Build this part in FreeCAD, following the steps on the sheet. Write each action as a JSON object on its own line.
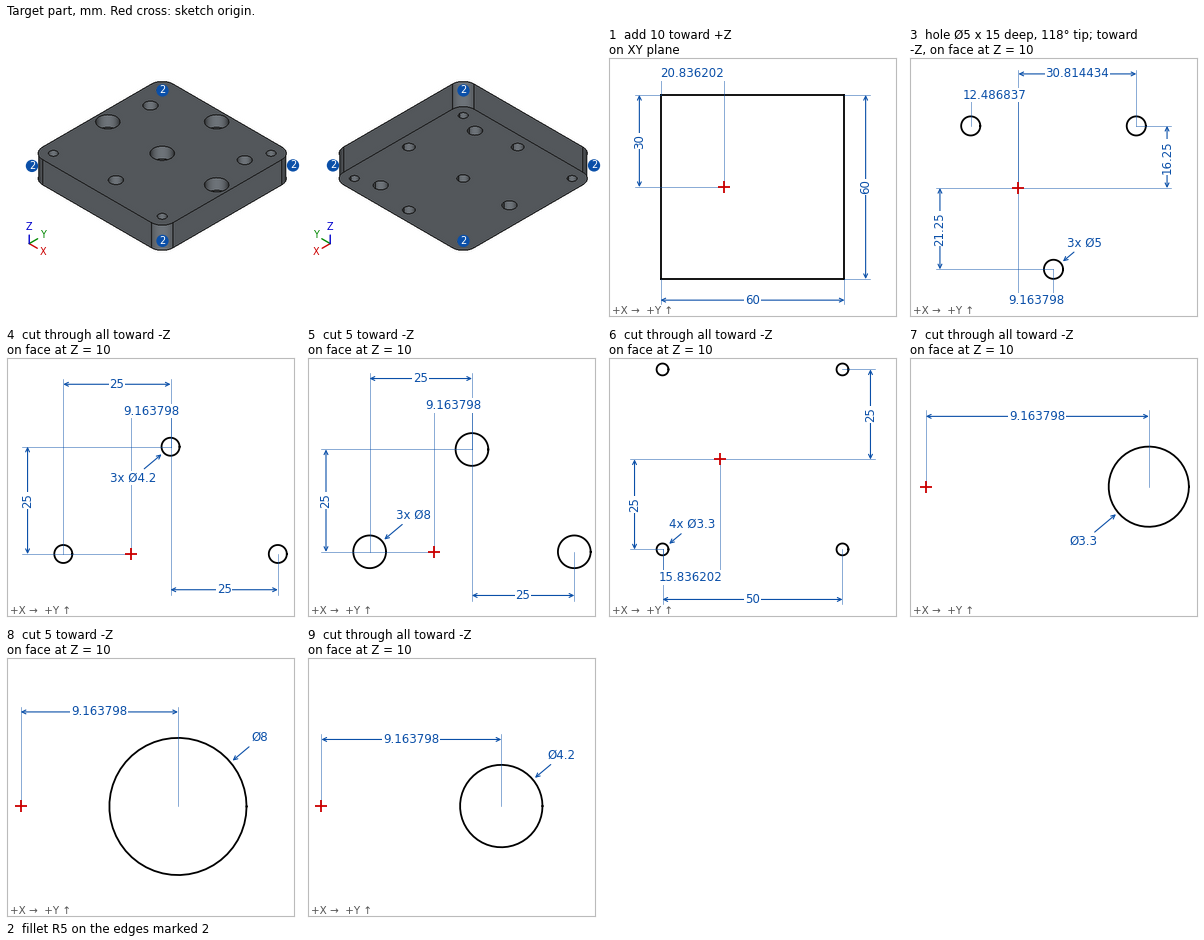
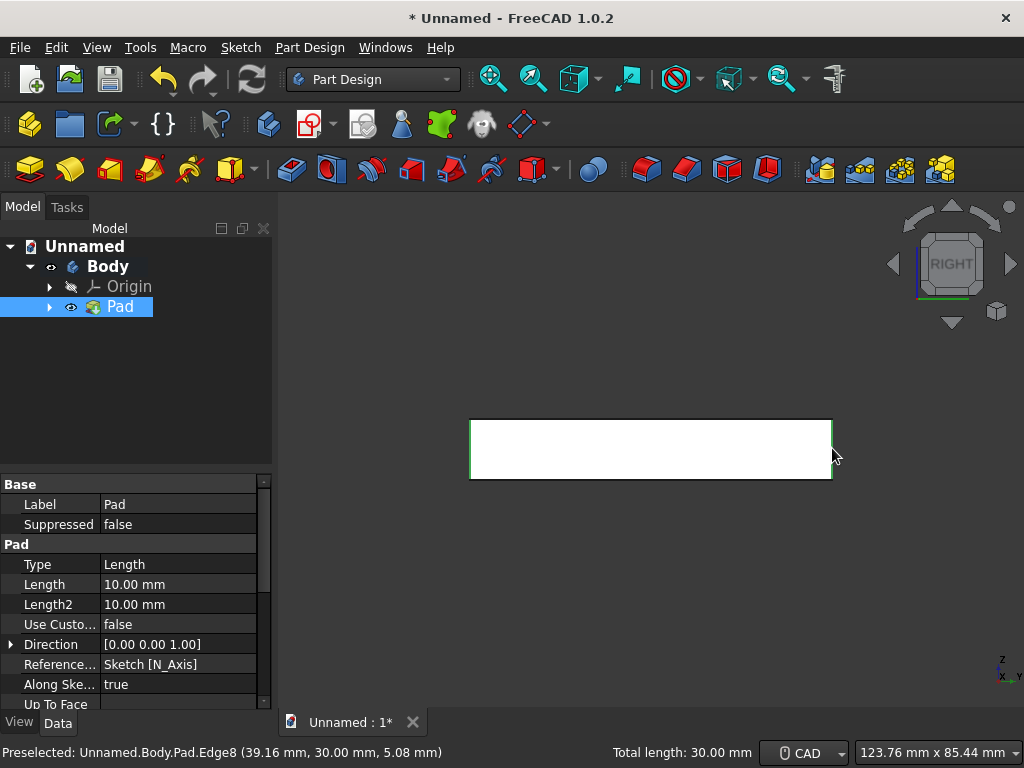
{"action": "key", "text": "5"}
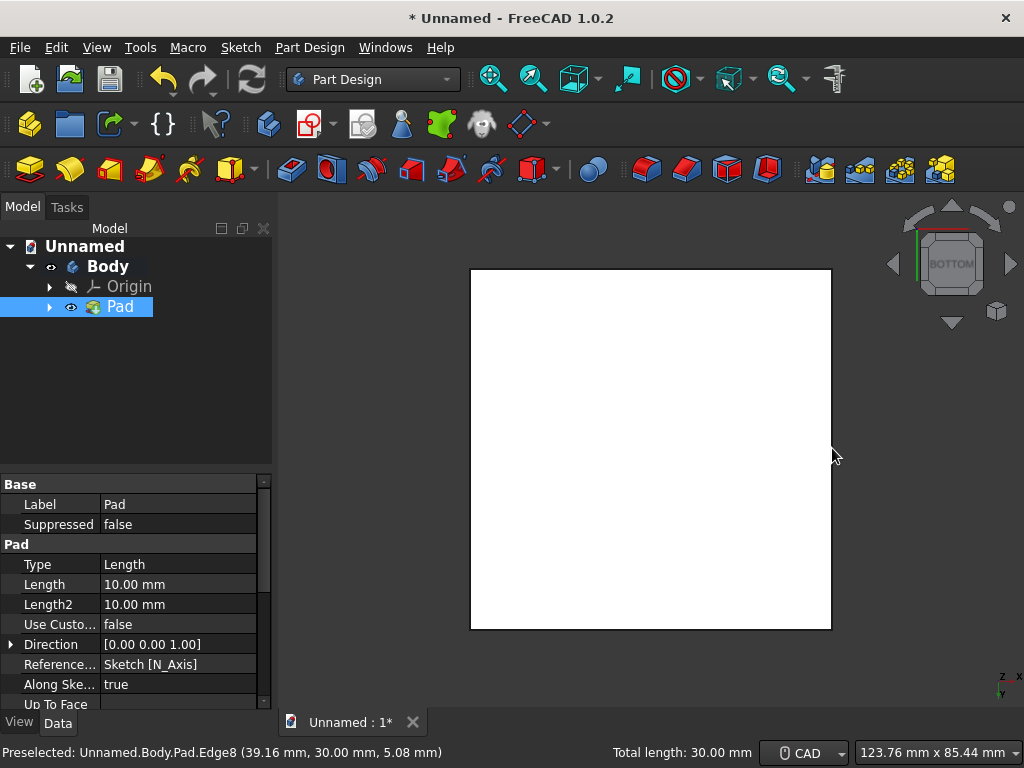
{"action": "key", "text": "4"}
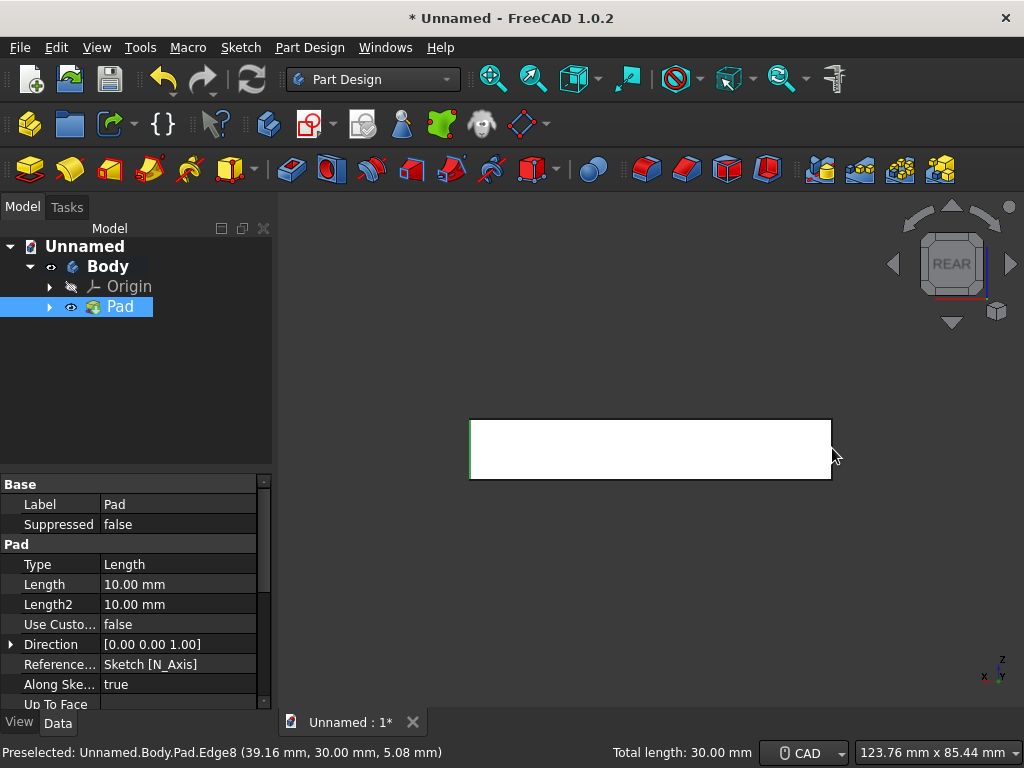
{"action": "left_click", "coordinate": [832, 449], "text": "ctrl"}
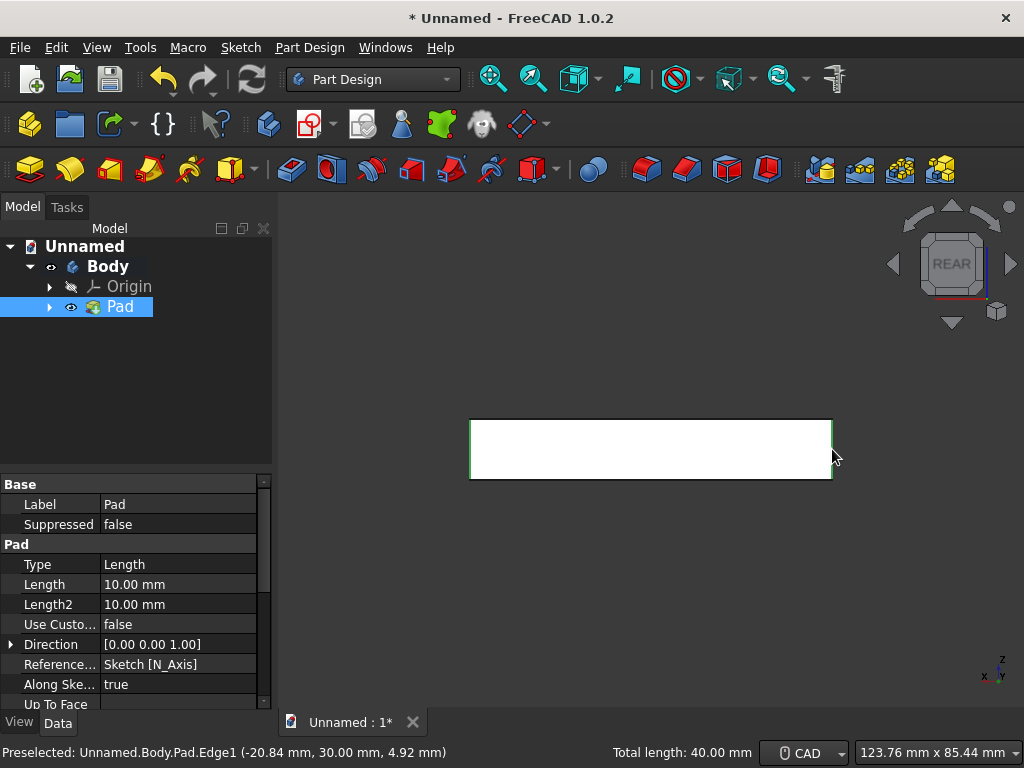
{"action": "left_click", "coordinate": [648, 170]}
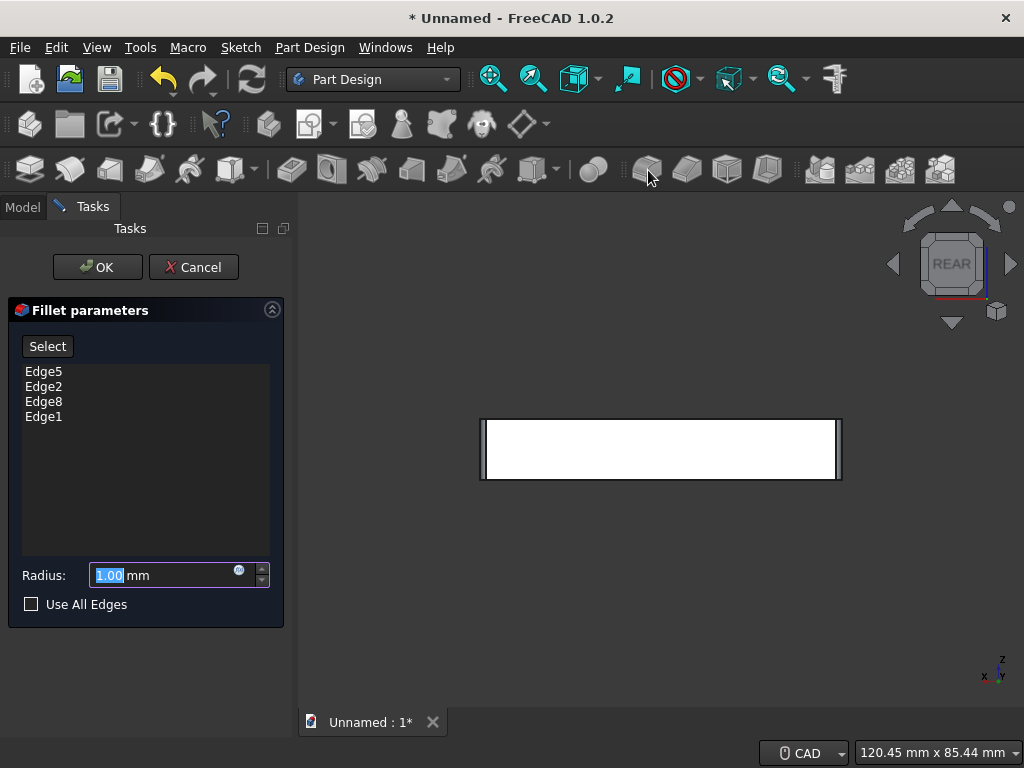
{"action": "type", "text": "5"}
{"action": "key", "text": "Tab"}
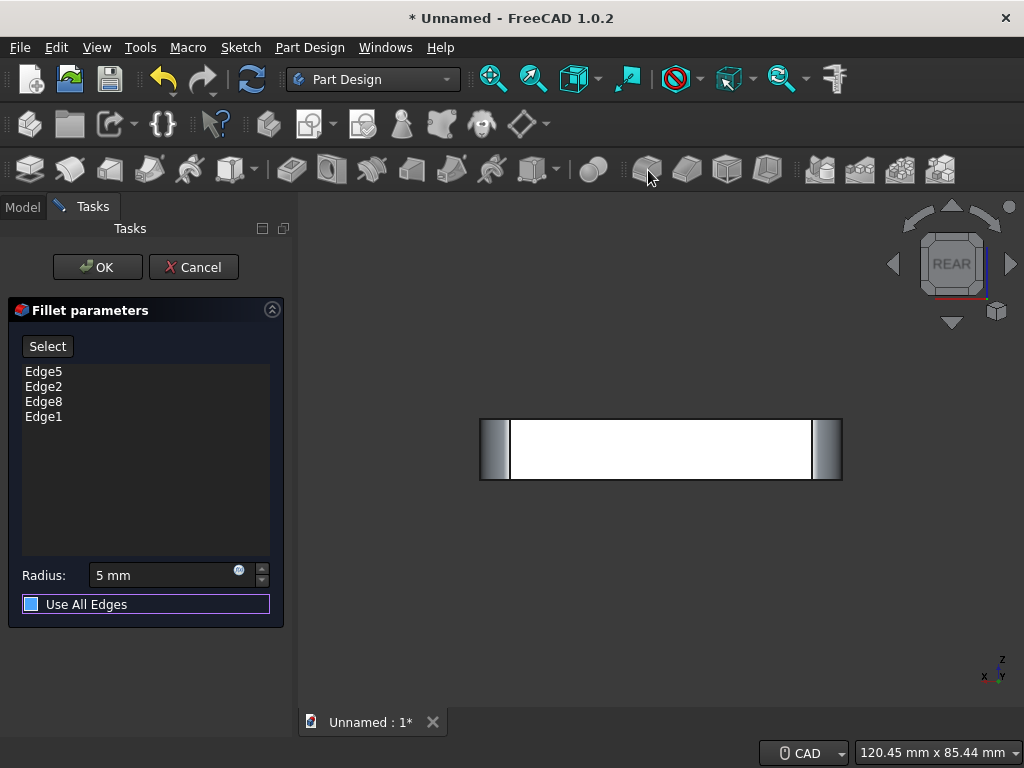
{"action": "left_click", "coordinate": [98, 267]}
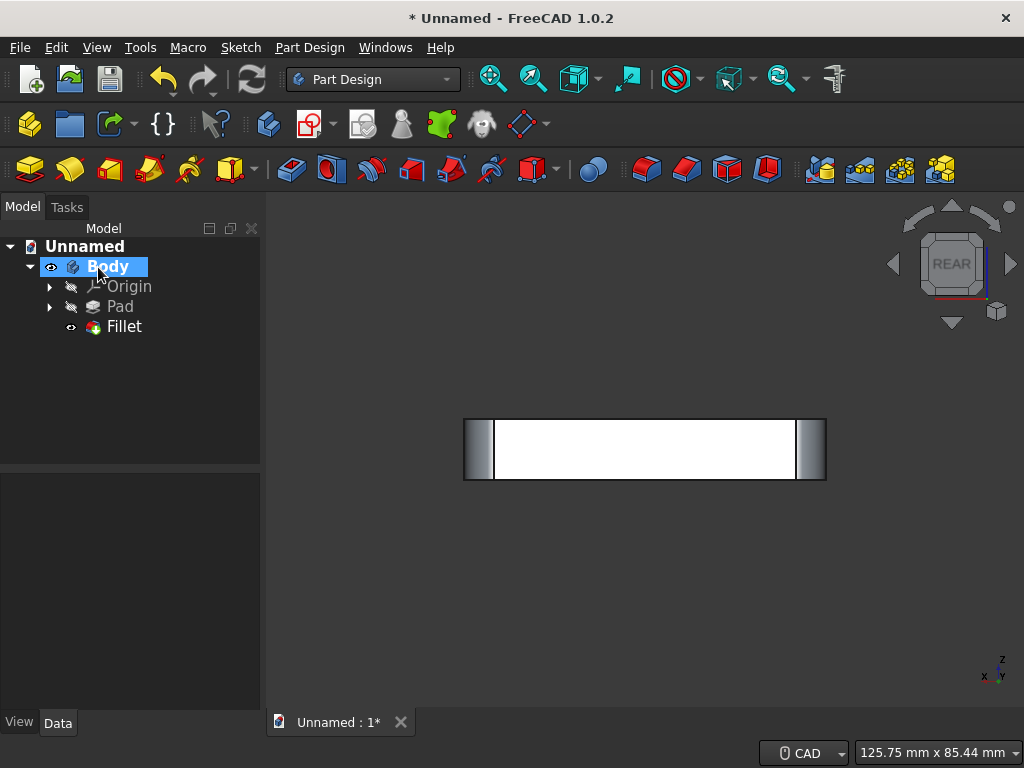
{"action": "key", "text": "0"}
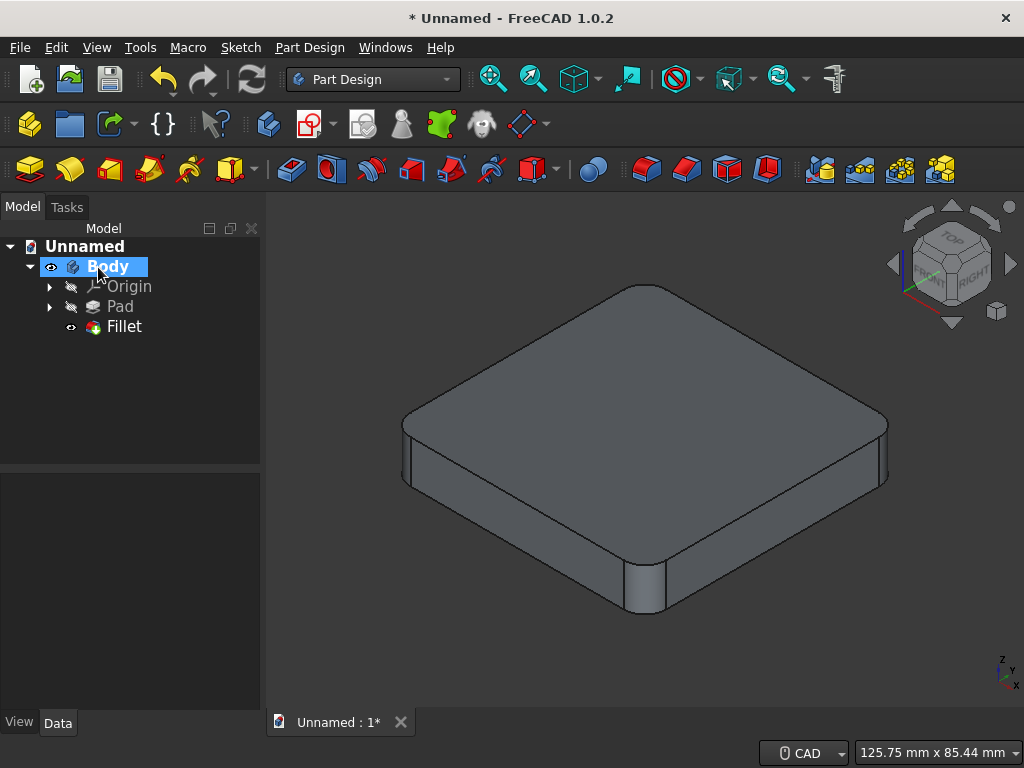
{"action": "left_click", "coordinate": [645, 424]}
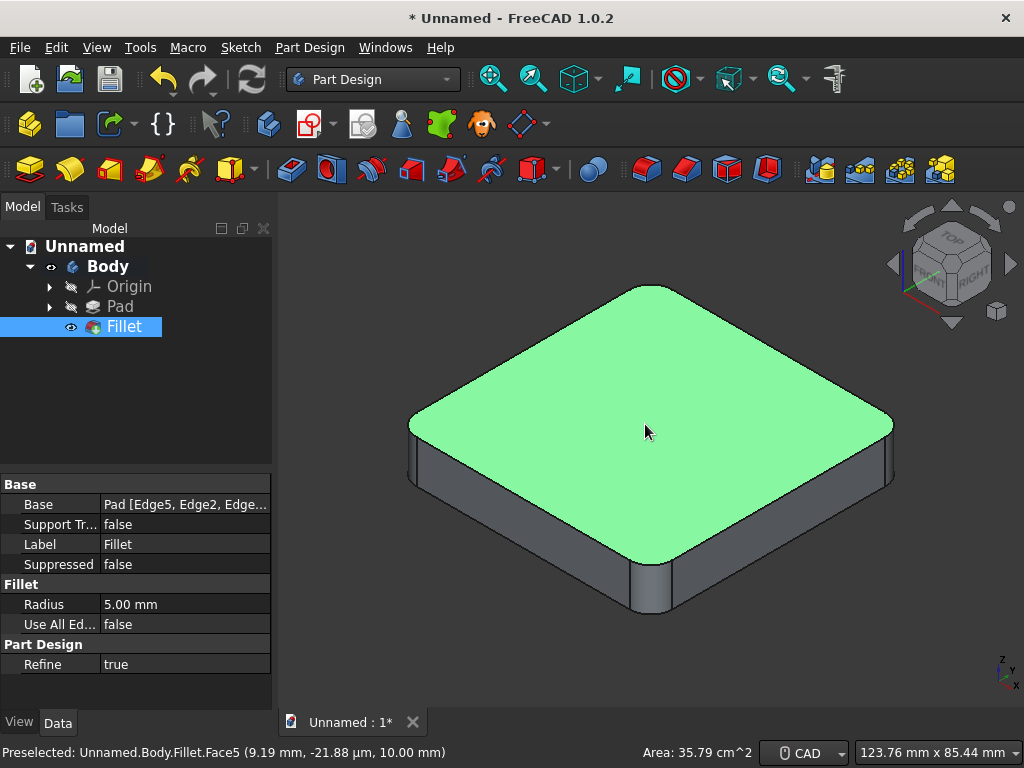
{"action": "left_click", "coordinate": [310, 124]}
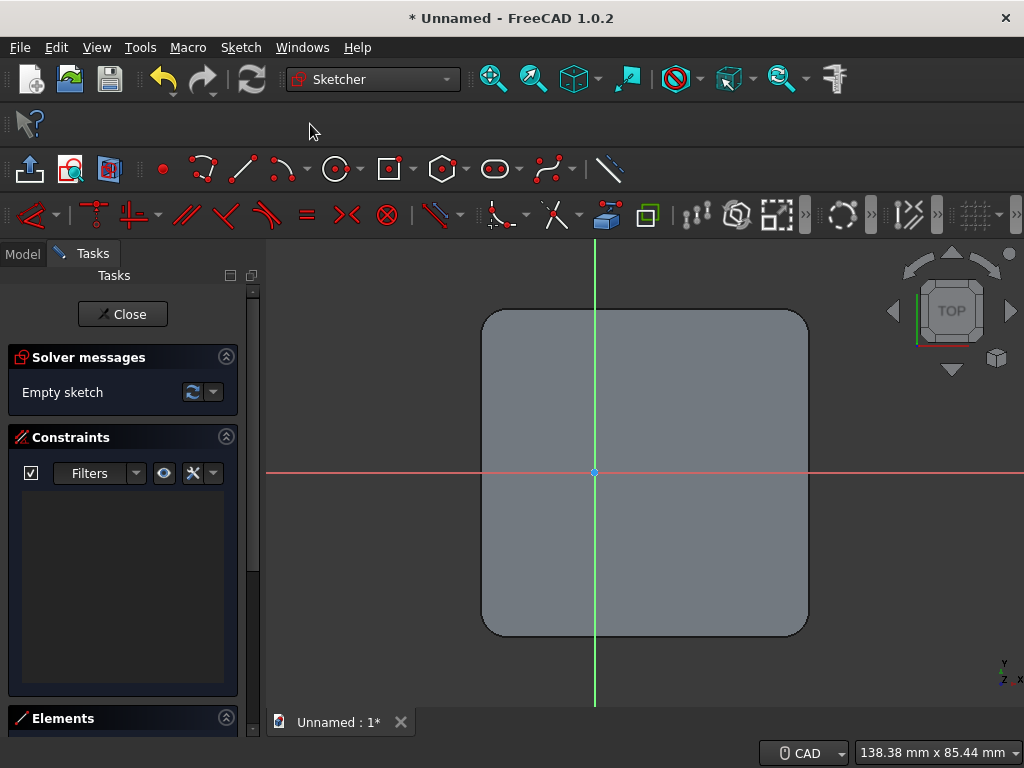
{"action": "left_click", "coordinate": [336, 170]}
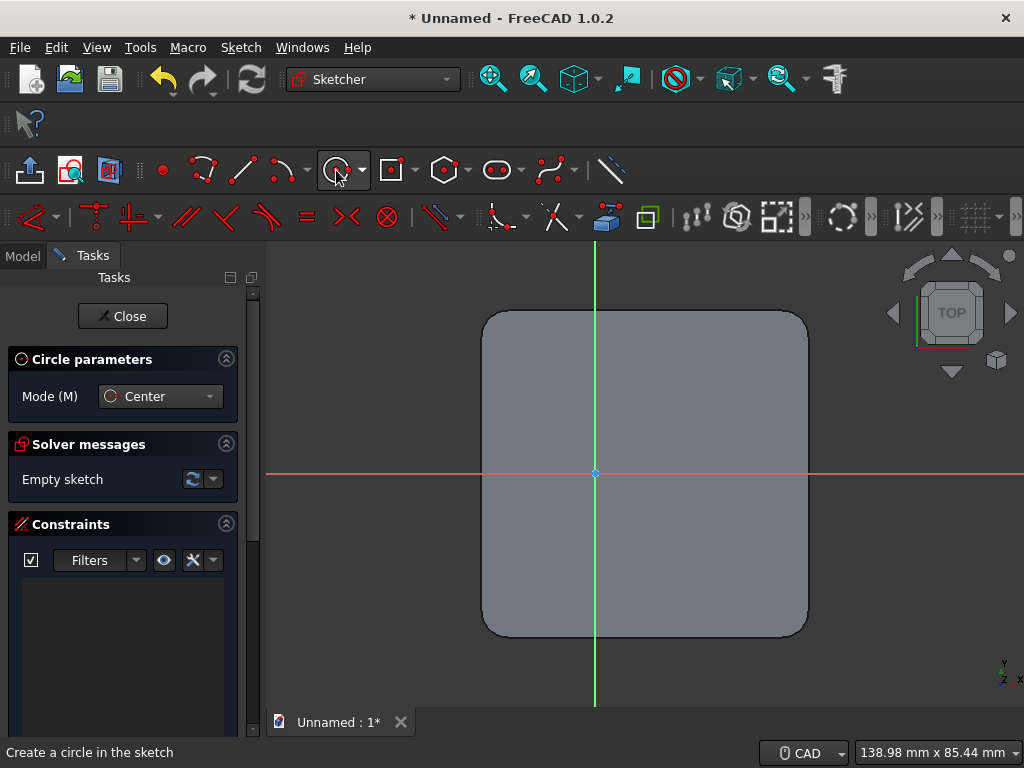
{"action": "scroll", "coordinate": [645, 590], "scroll_direction": "up", "scroll_amount": 3}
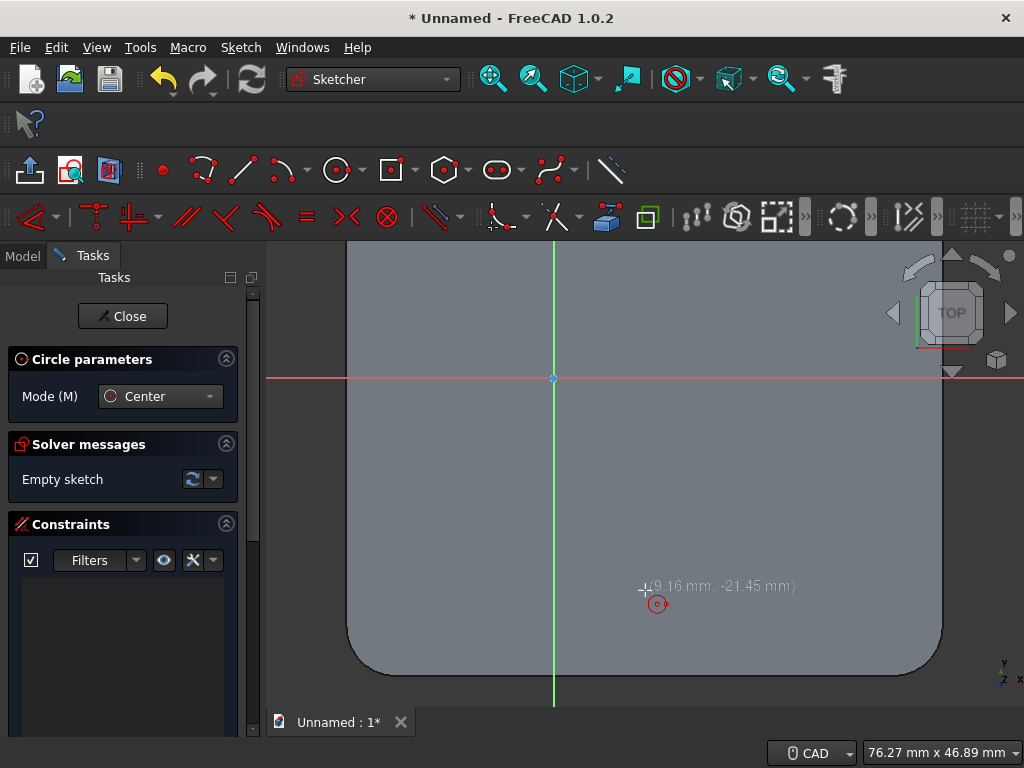
{"action": "left_click", "coordinate": [645, 589]}
{"action": "mouse_move", "coordinate": [662, 572]}